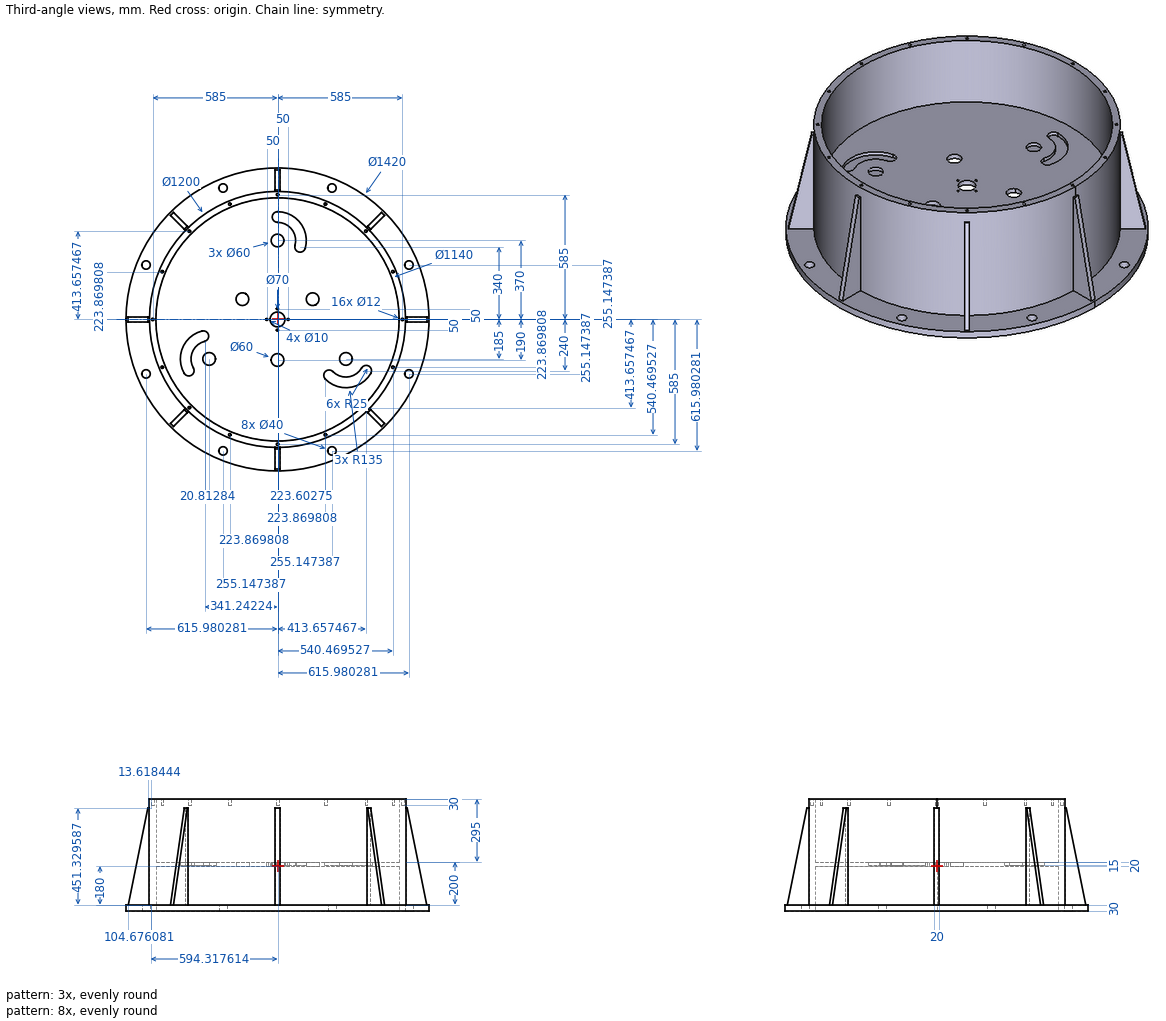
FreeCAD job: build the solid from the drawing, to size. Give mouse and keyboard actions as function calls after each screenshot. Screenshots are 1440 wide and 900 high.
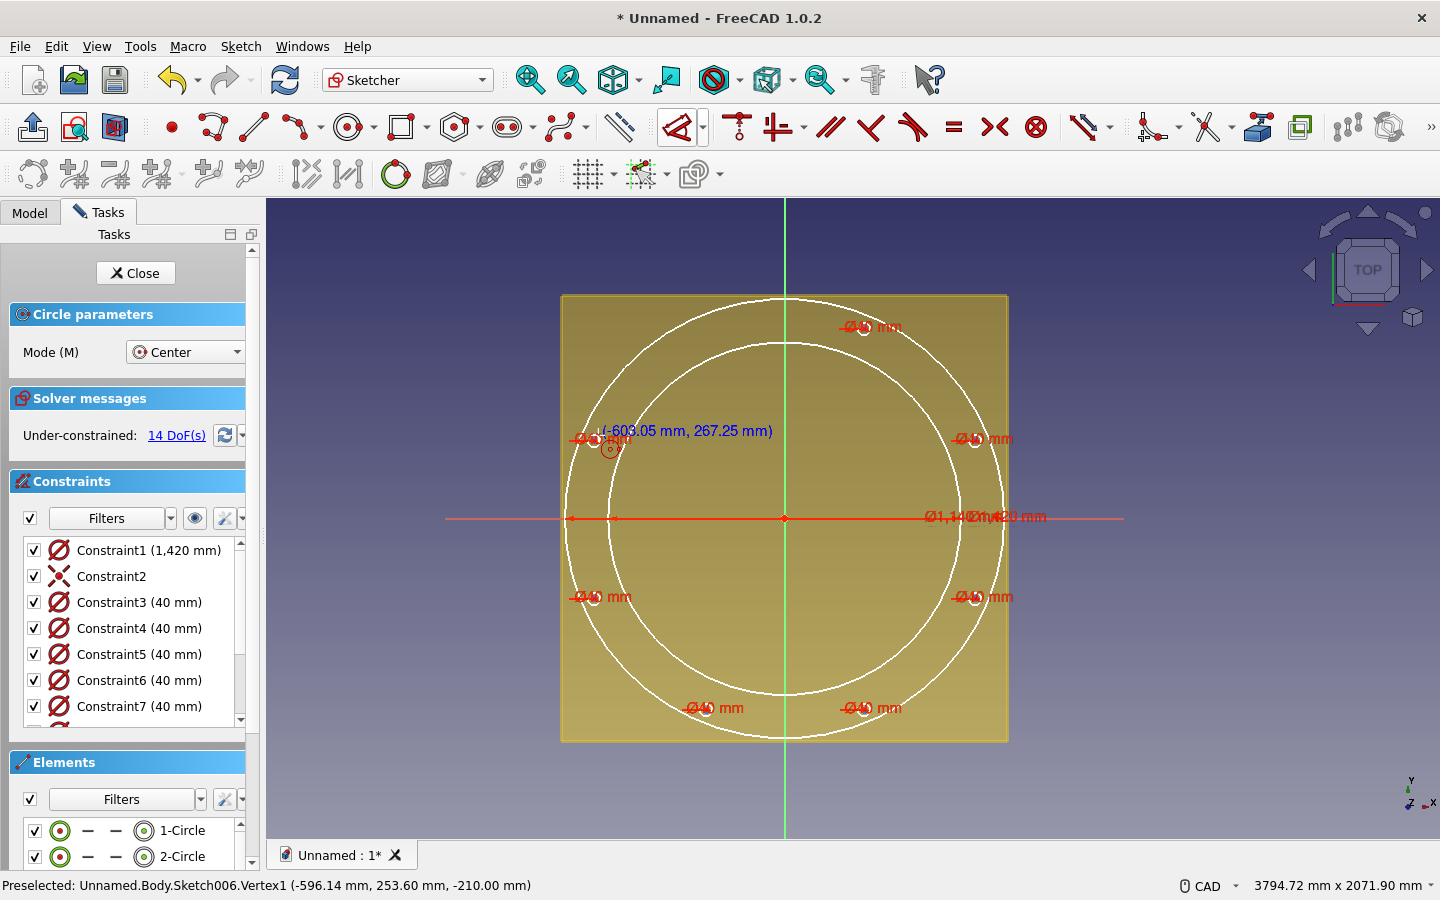
scroll(706, 328, up, 7)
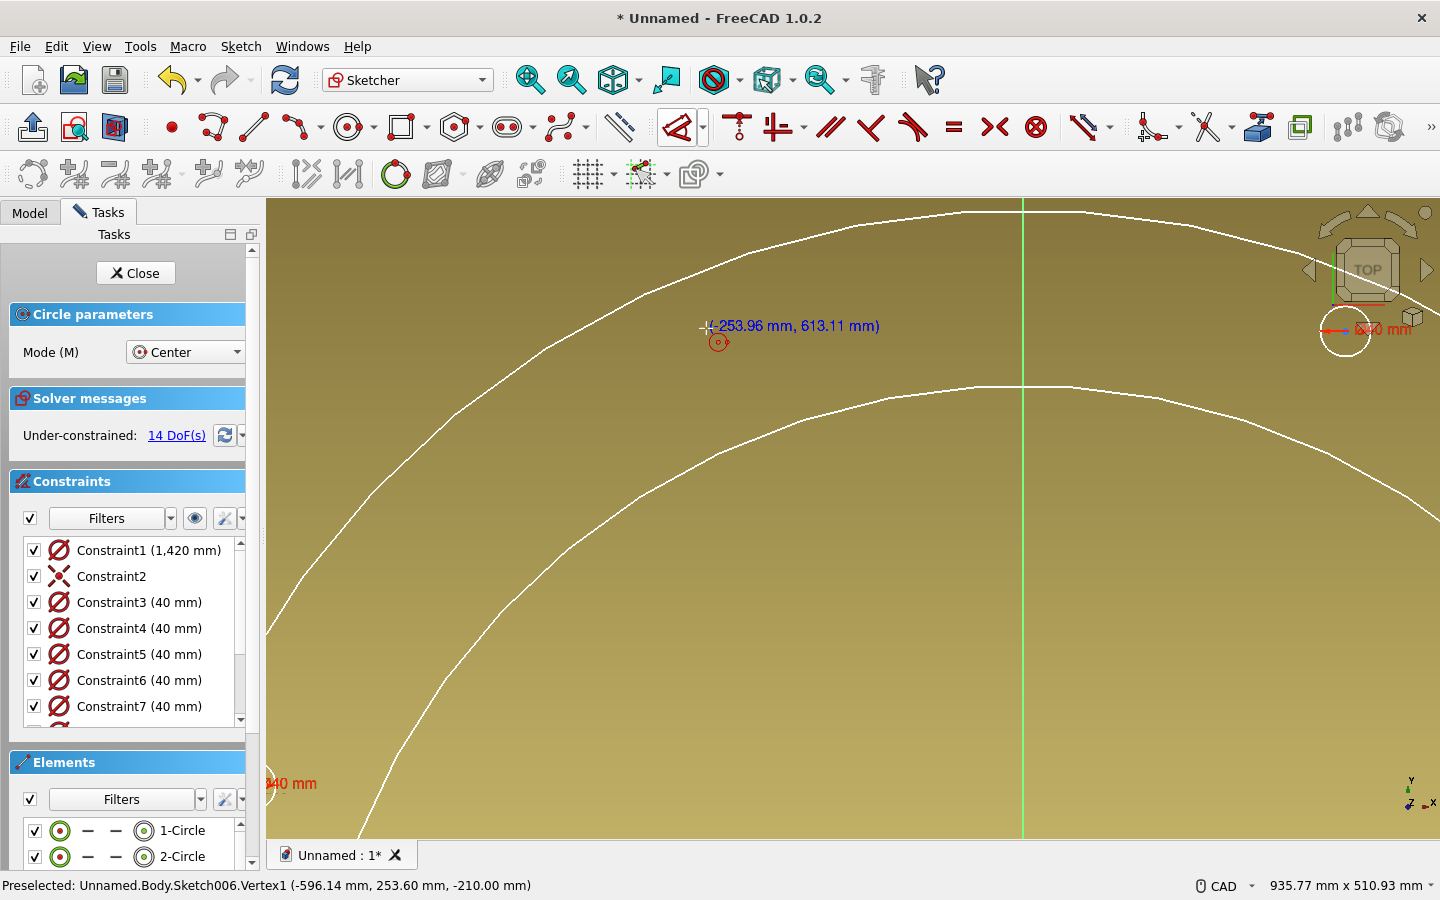
scroll(706, 328, down, 7)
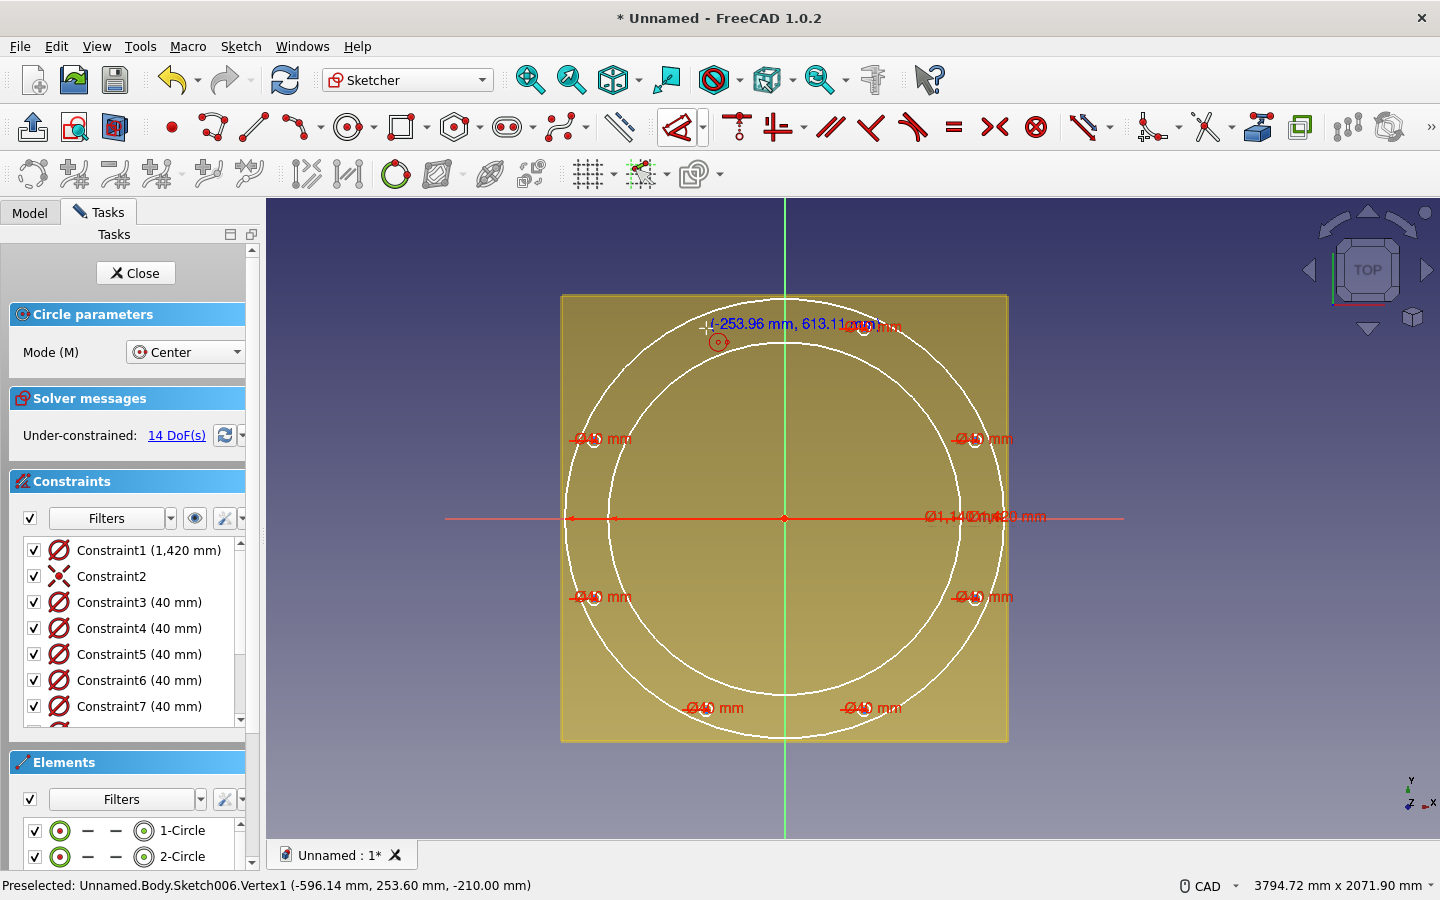
click(706, 328)
move(710, 332)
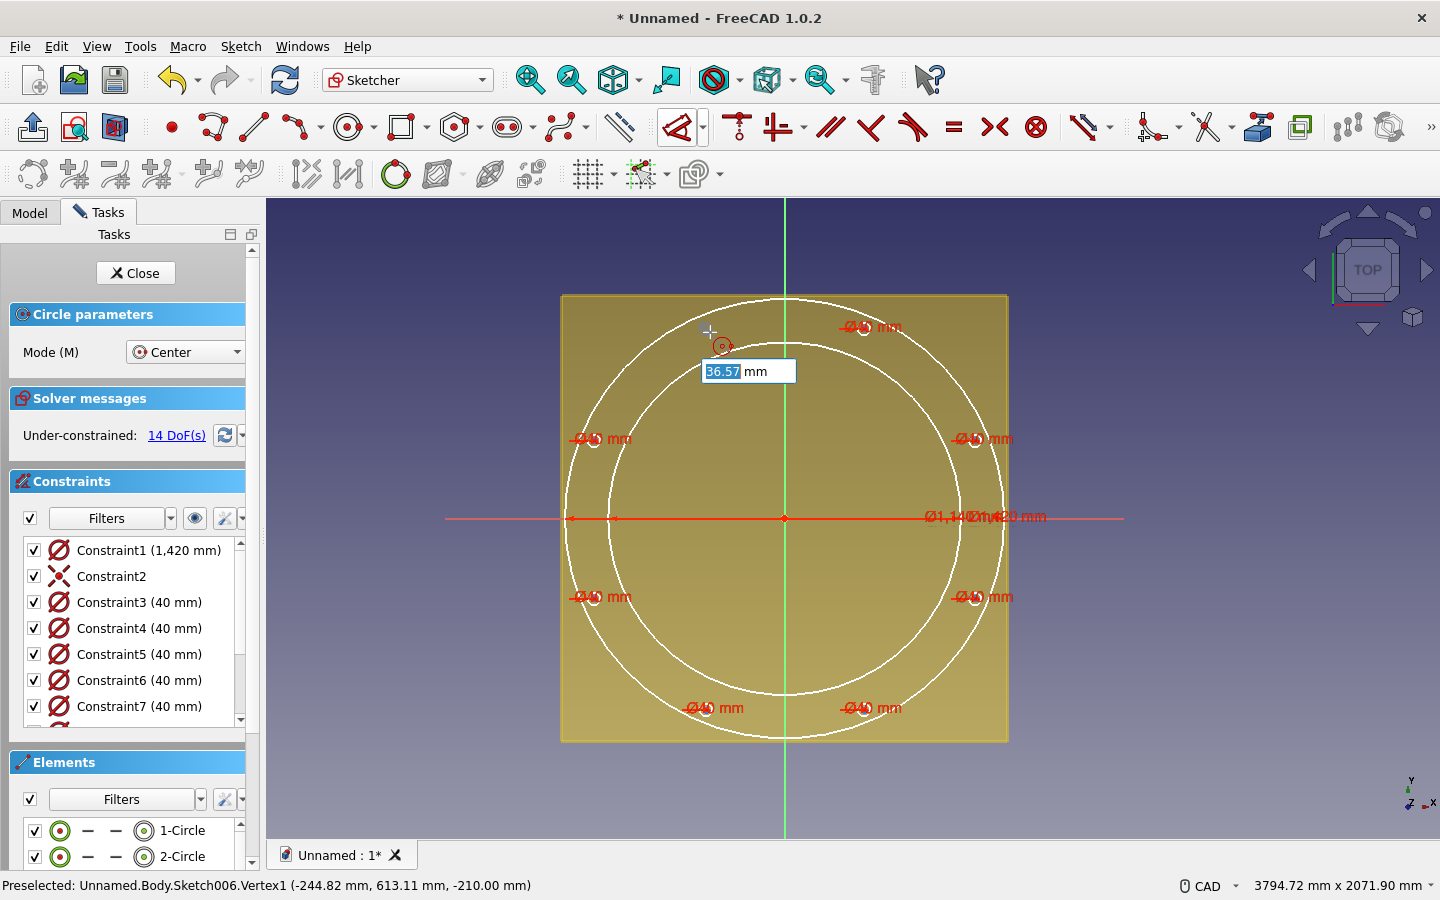
text(40)
key(Return)
key(Escape)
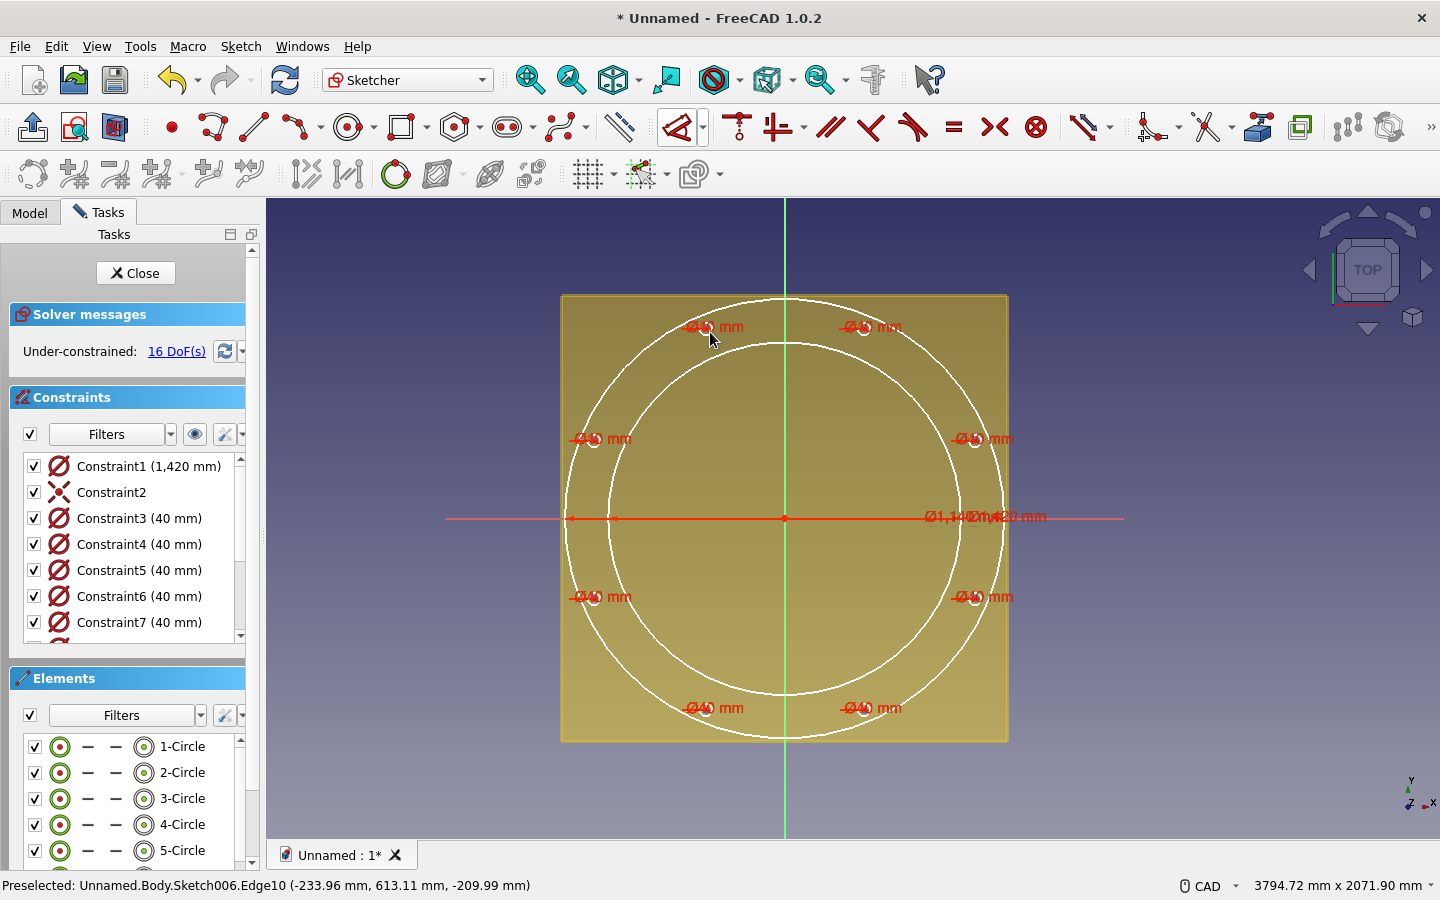
click(864, 710)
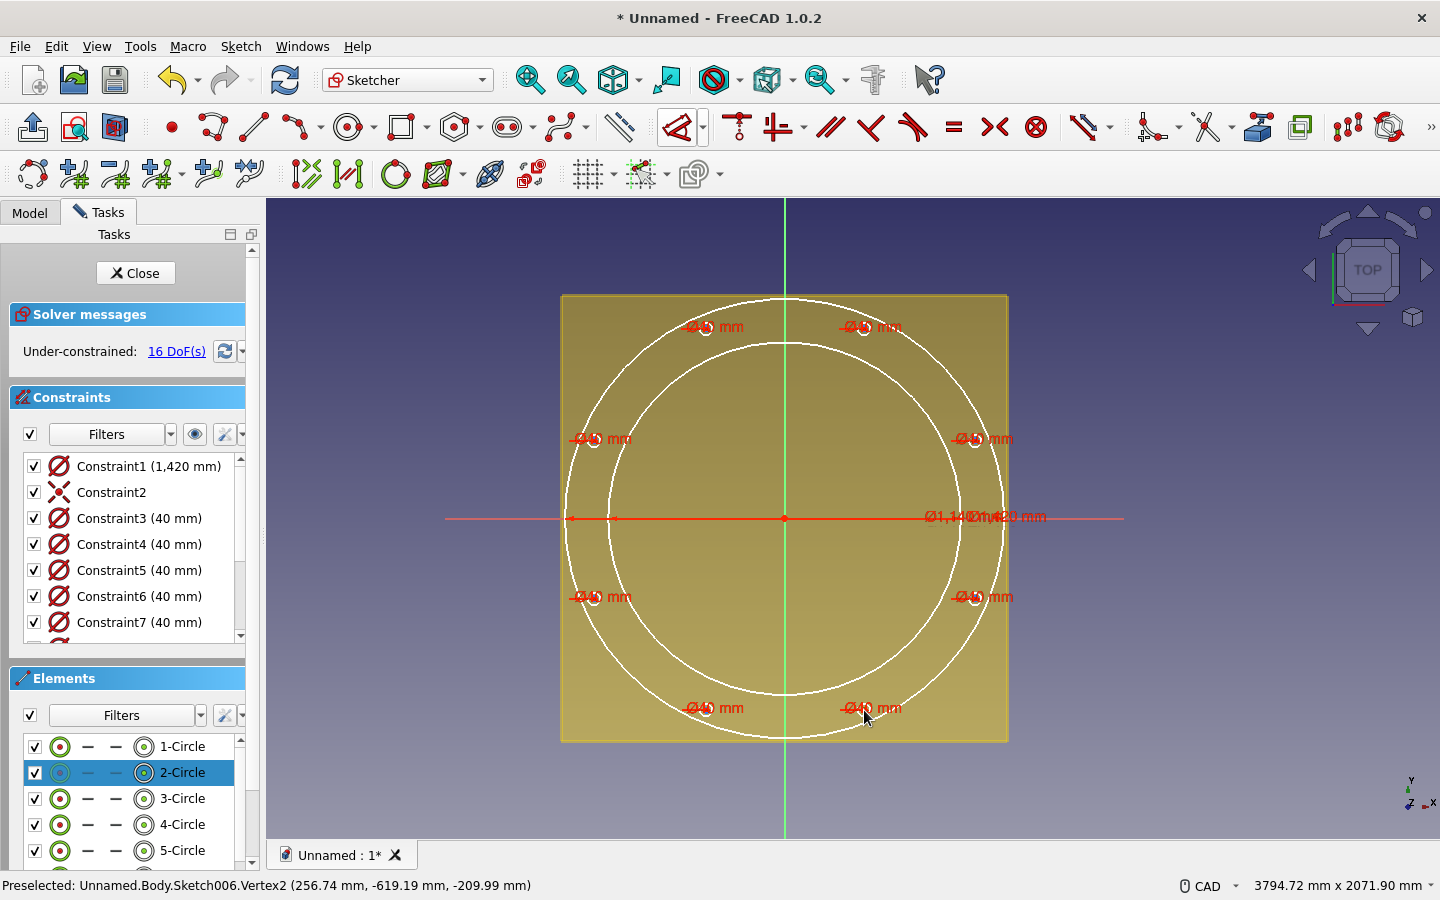
click(706, 710)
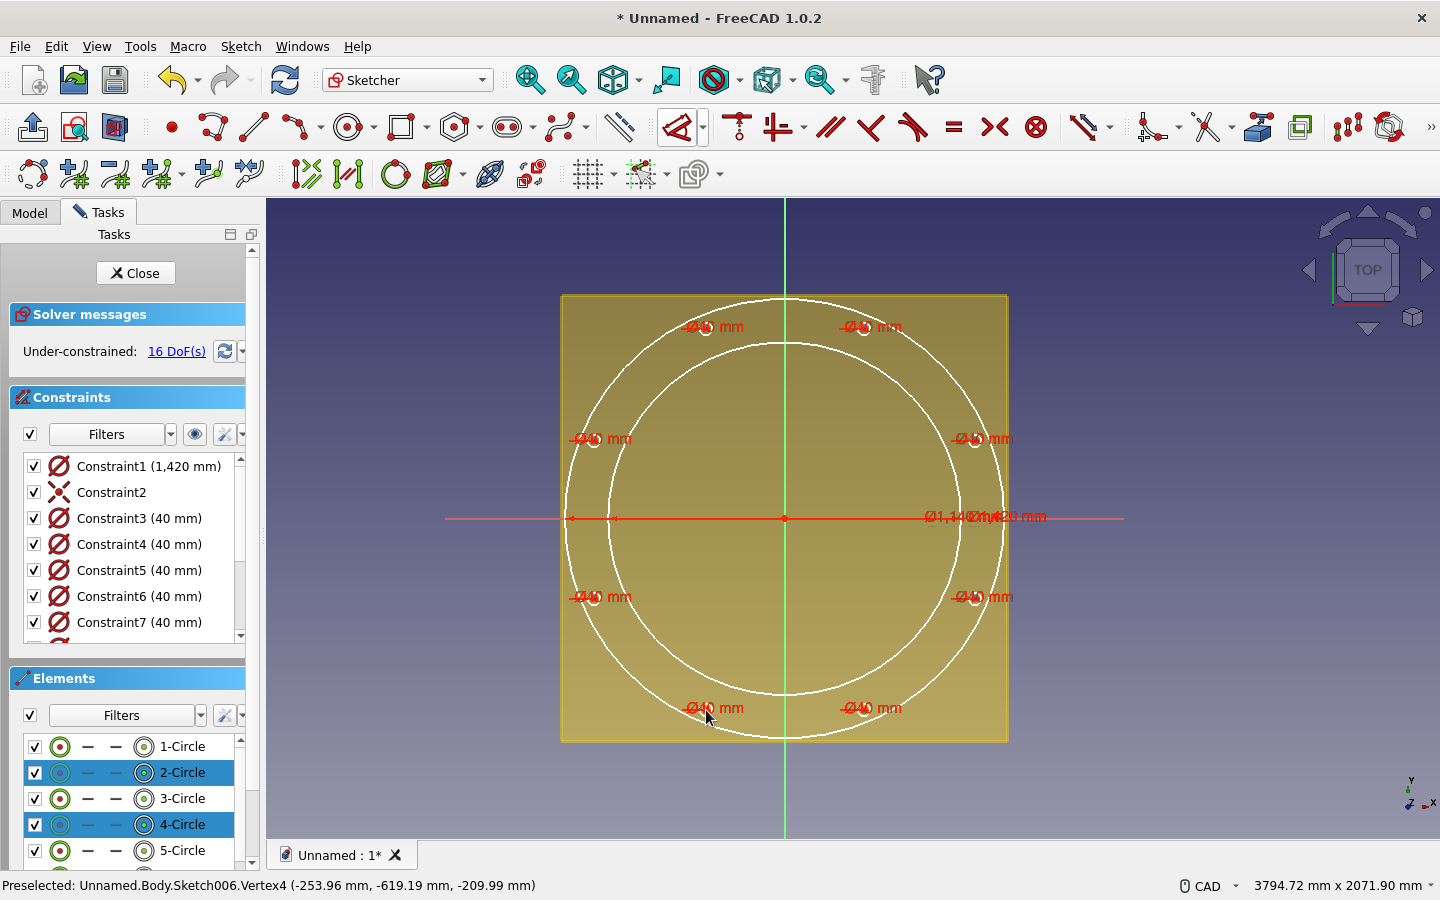
key(h)